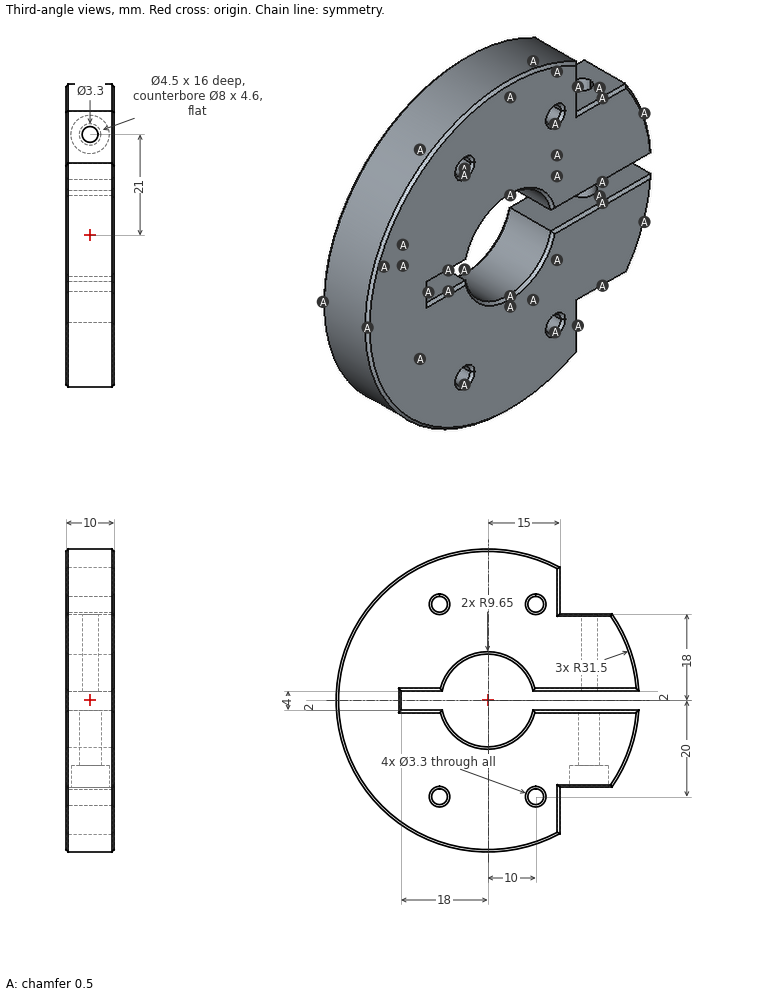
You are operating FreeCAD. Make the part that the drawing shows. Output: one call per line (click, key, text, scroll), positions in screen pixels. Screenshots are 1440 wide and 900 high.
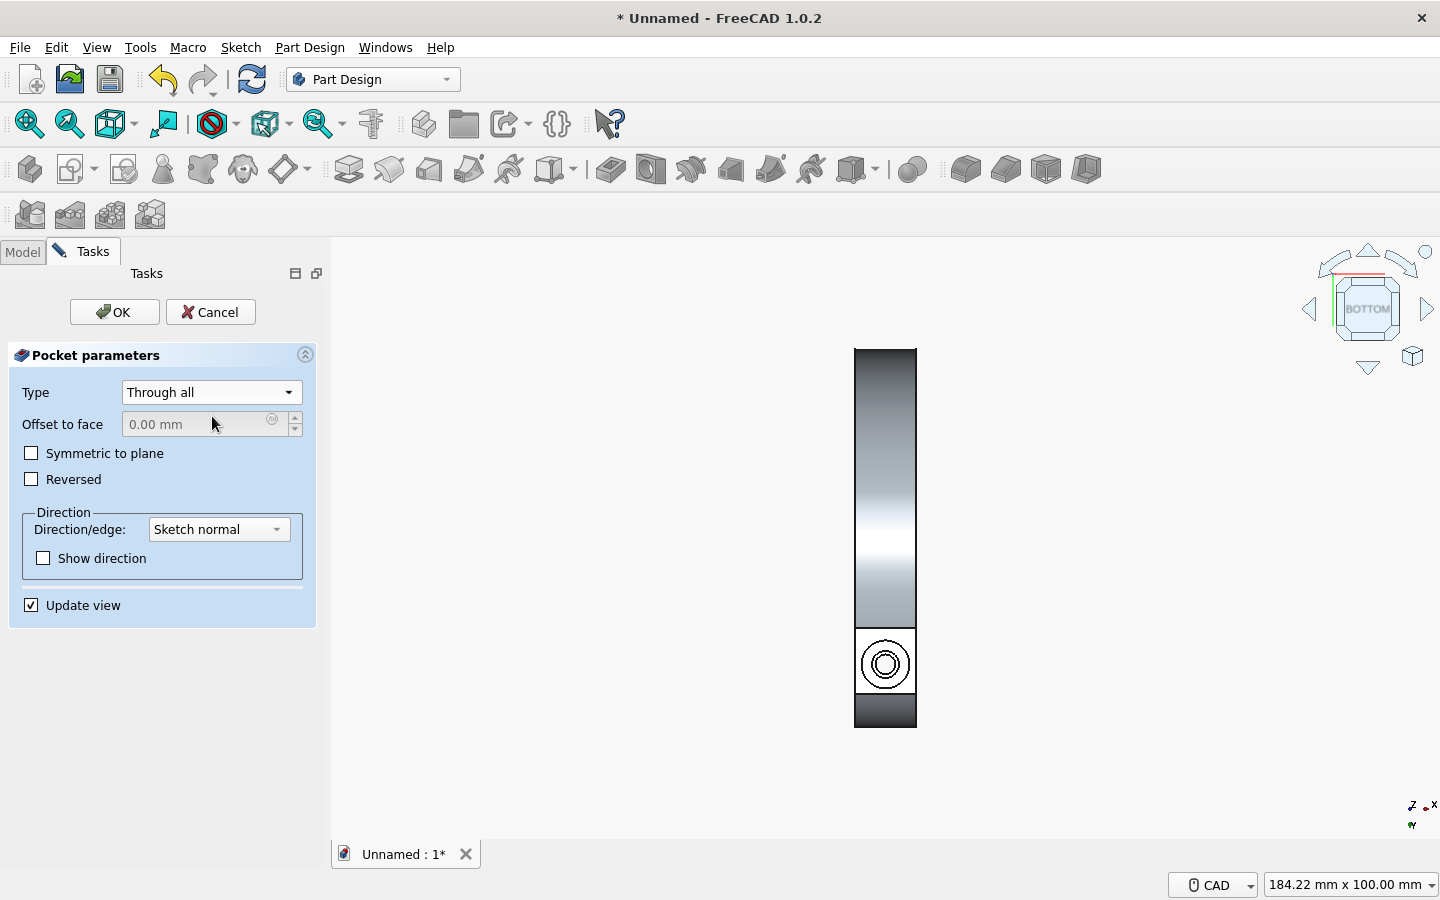
click(115, 312)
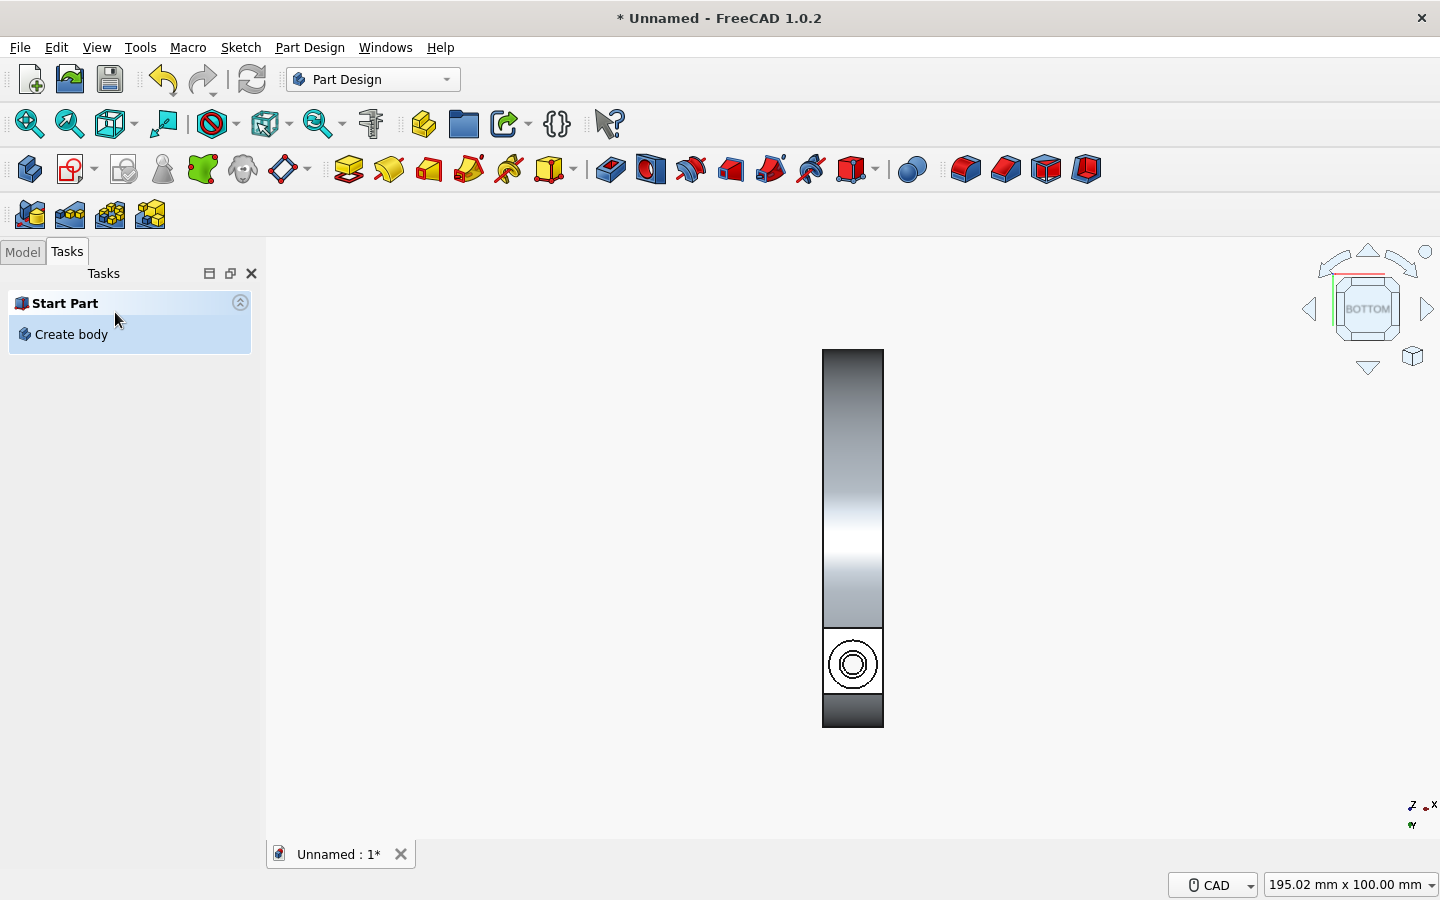
key(0)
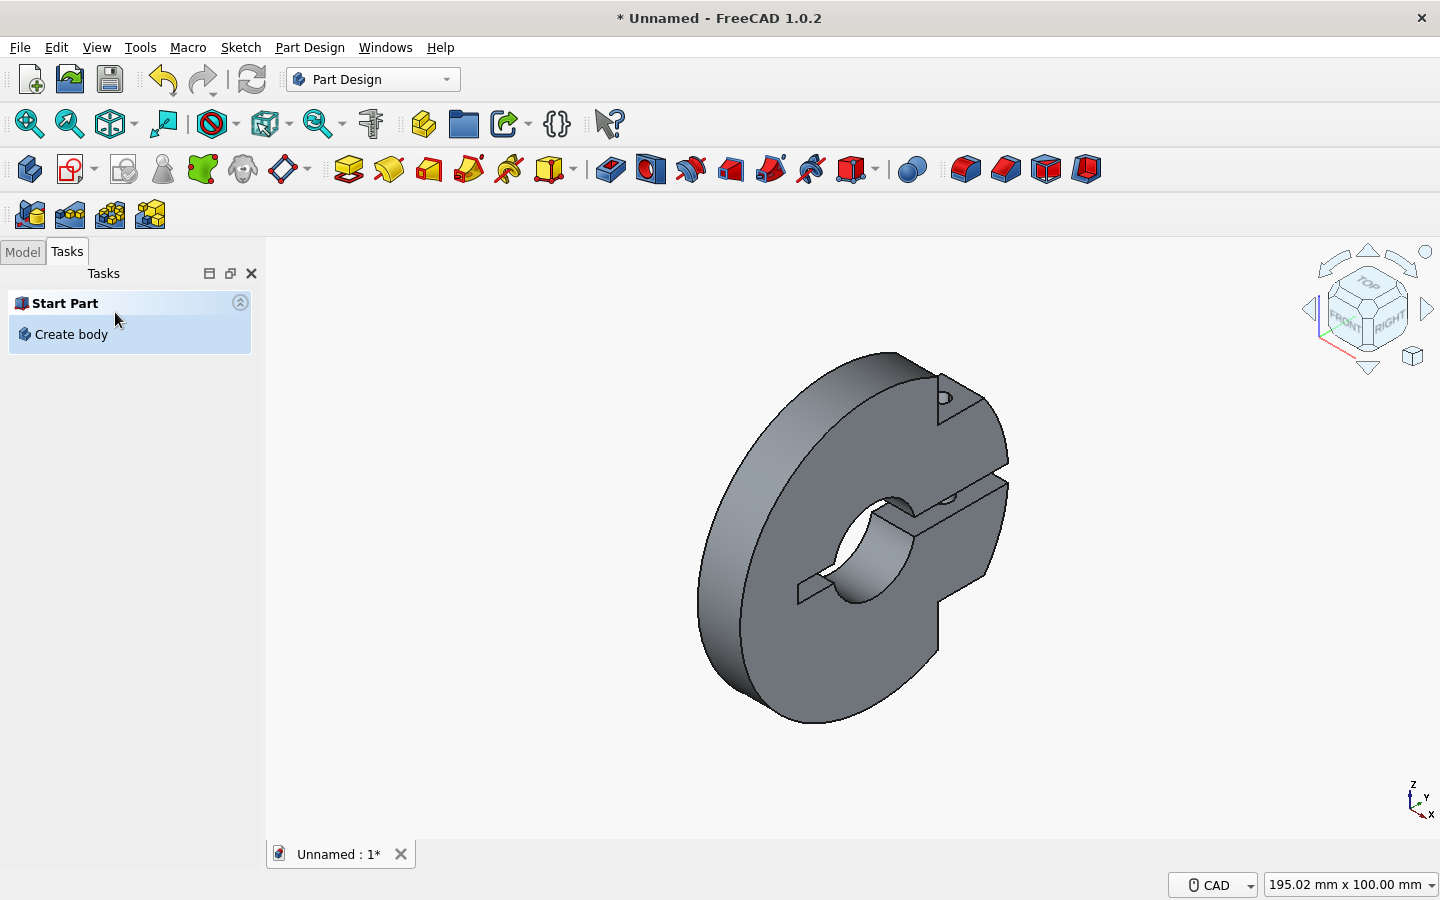
click(836, 483)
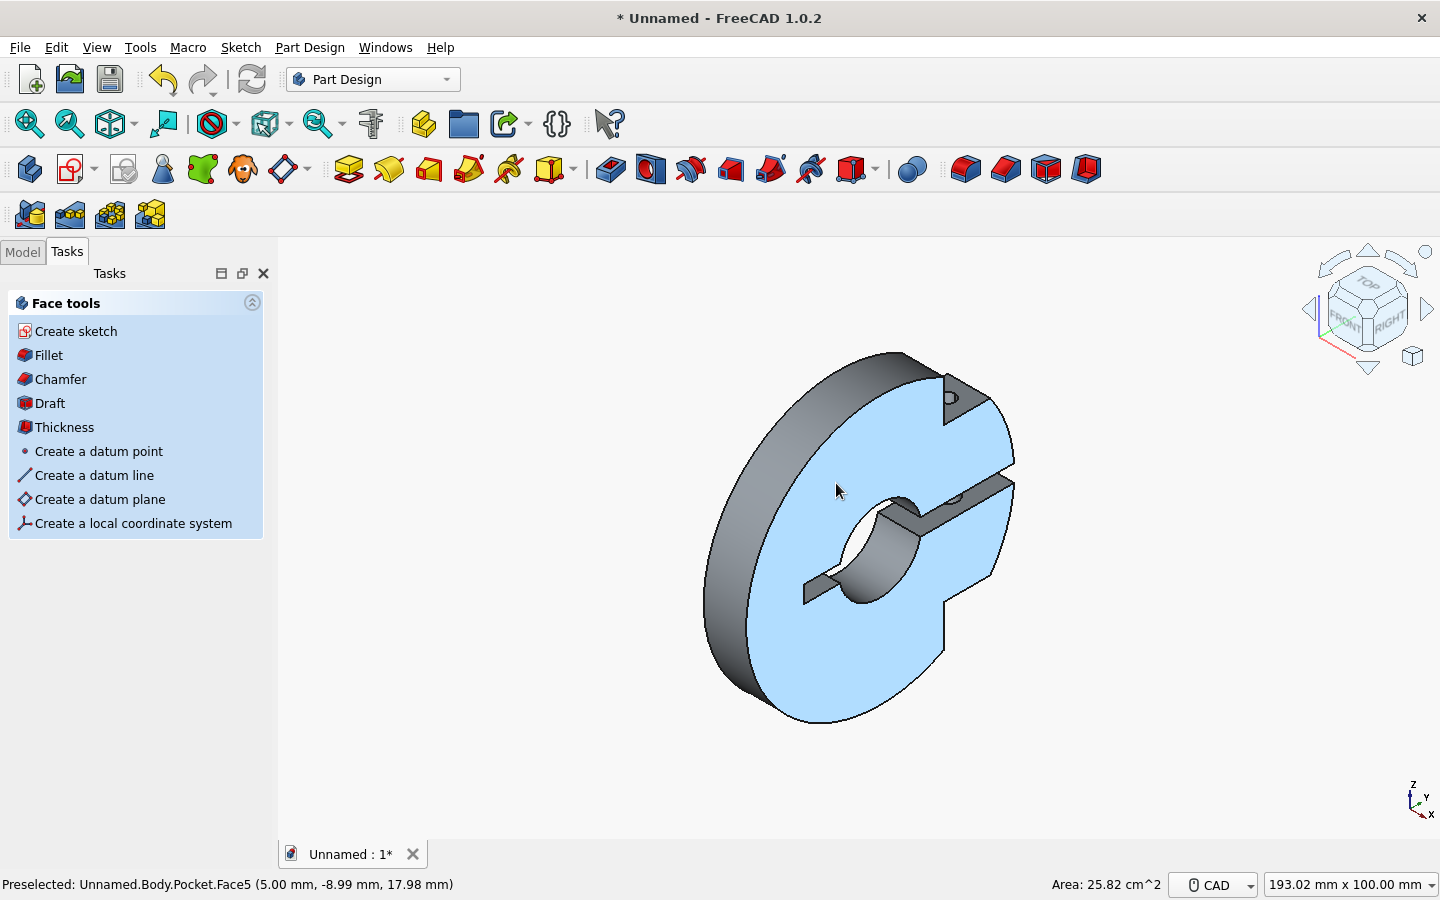
click(70, 170)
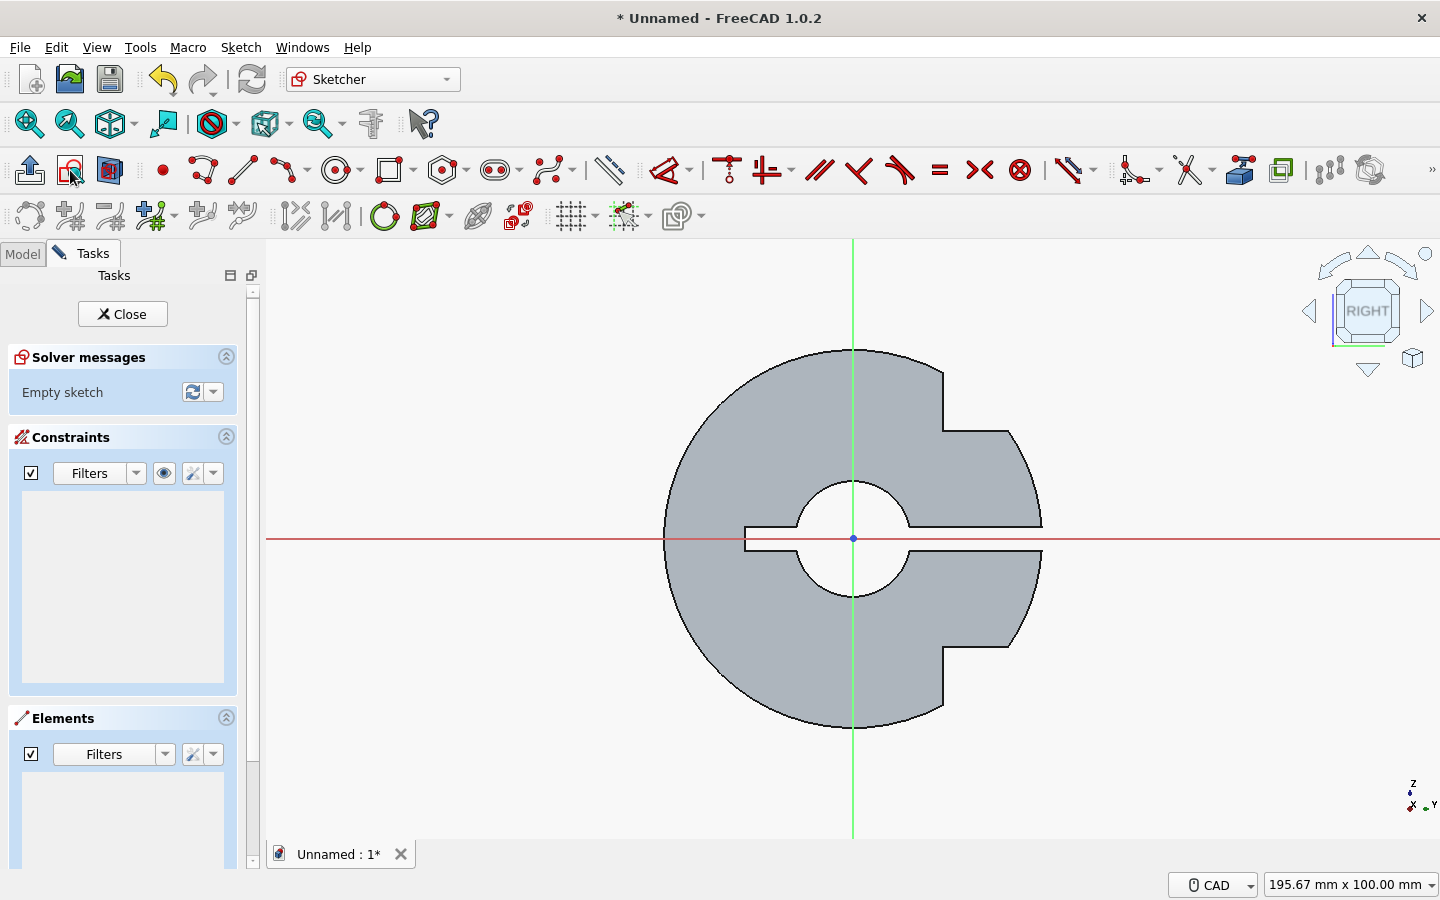
scroll(992, 539, up, 2)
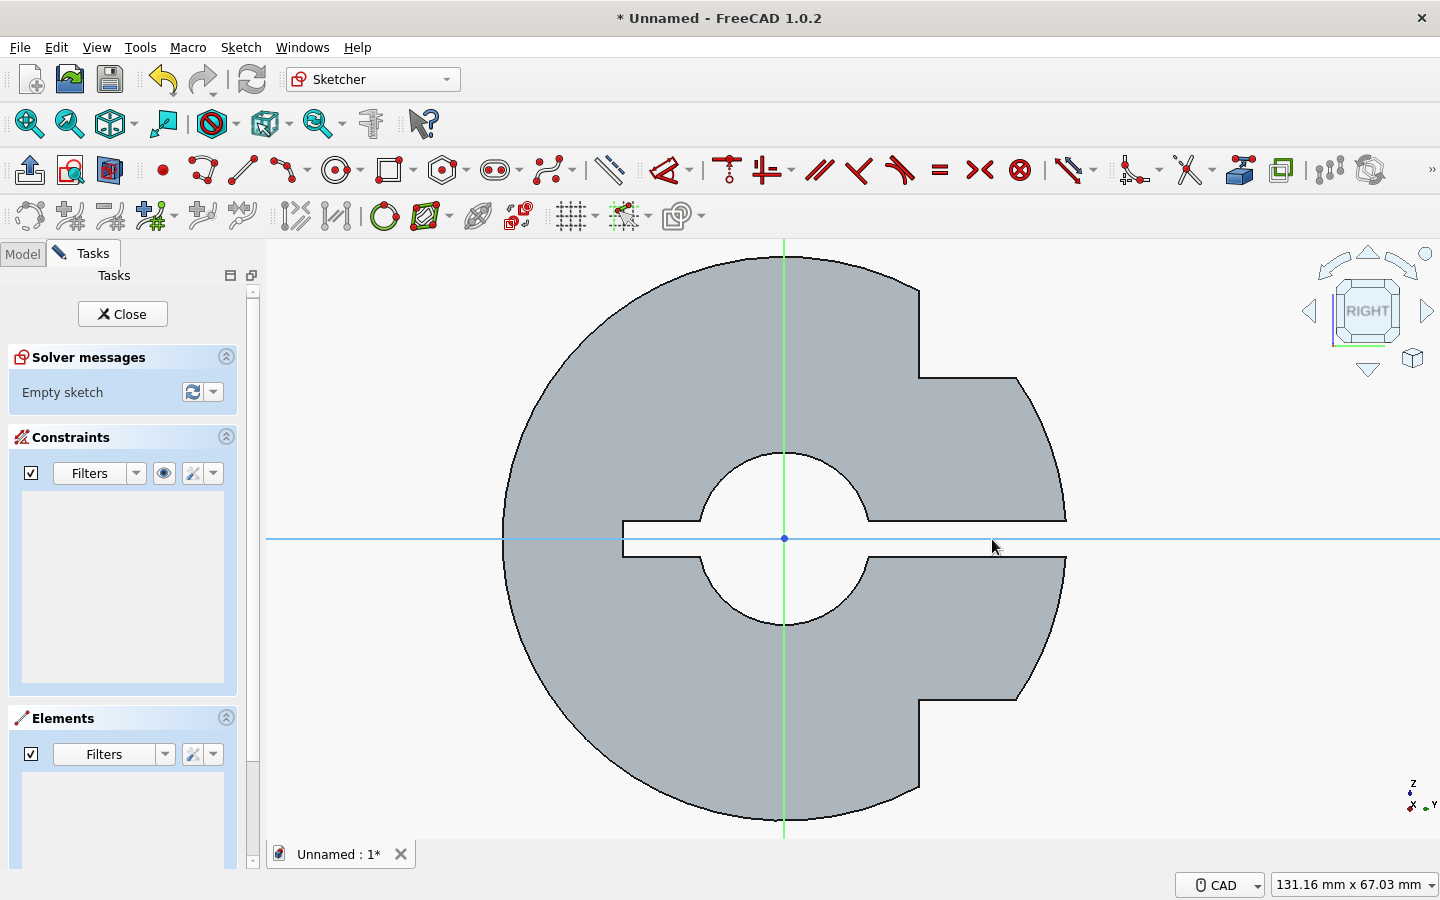
key(g)
key(c)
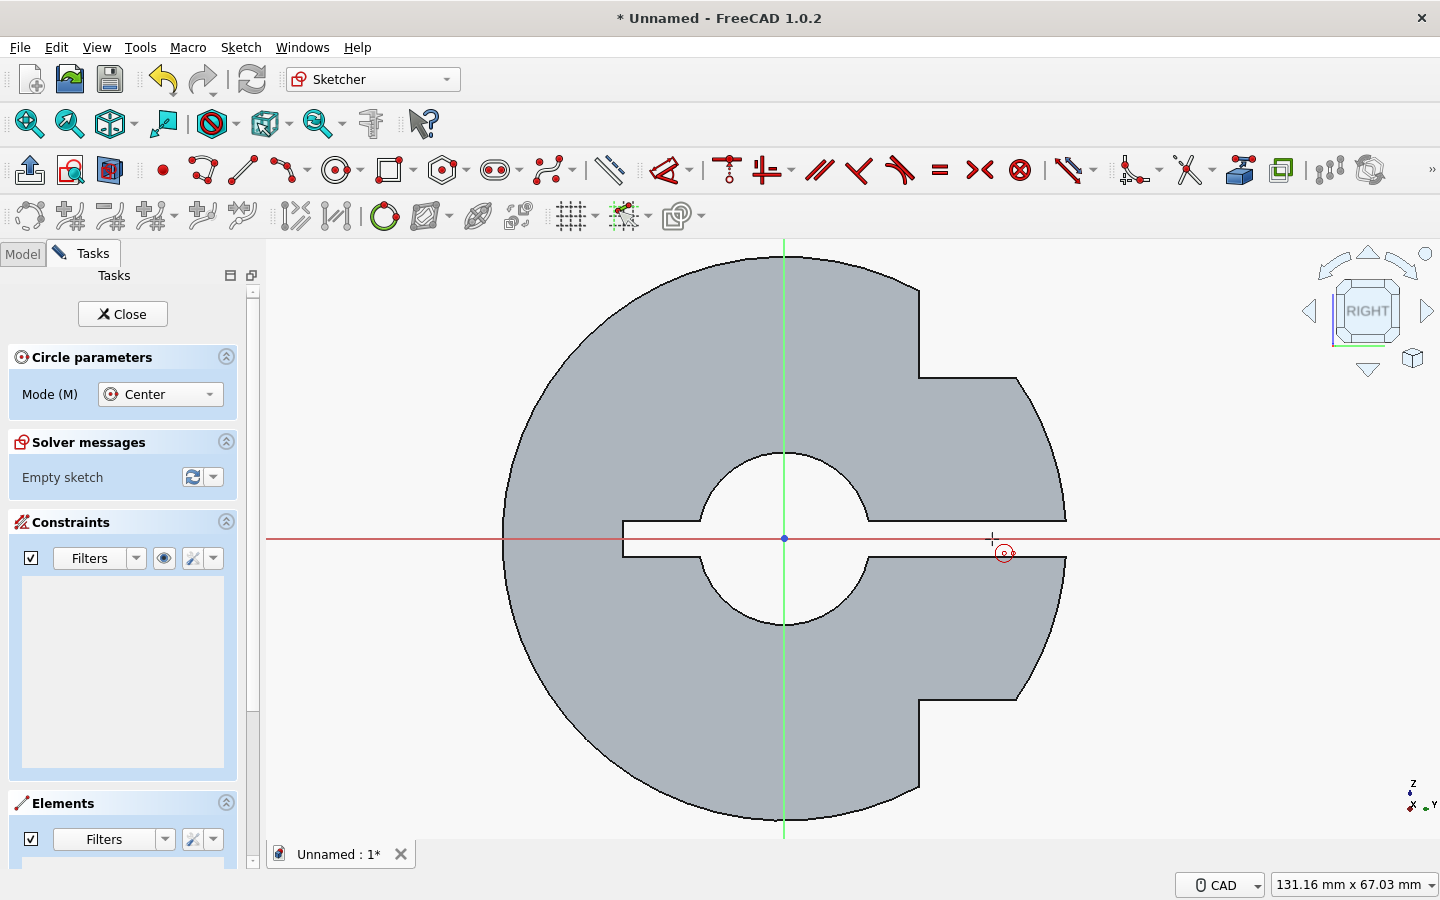
scroll(874, 718, up, 3)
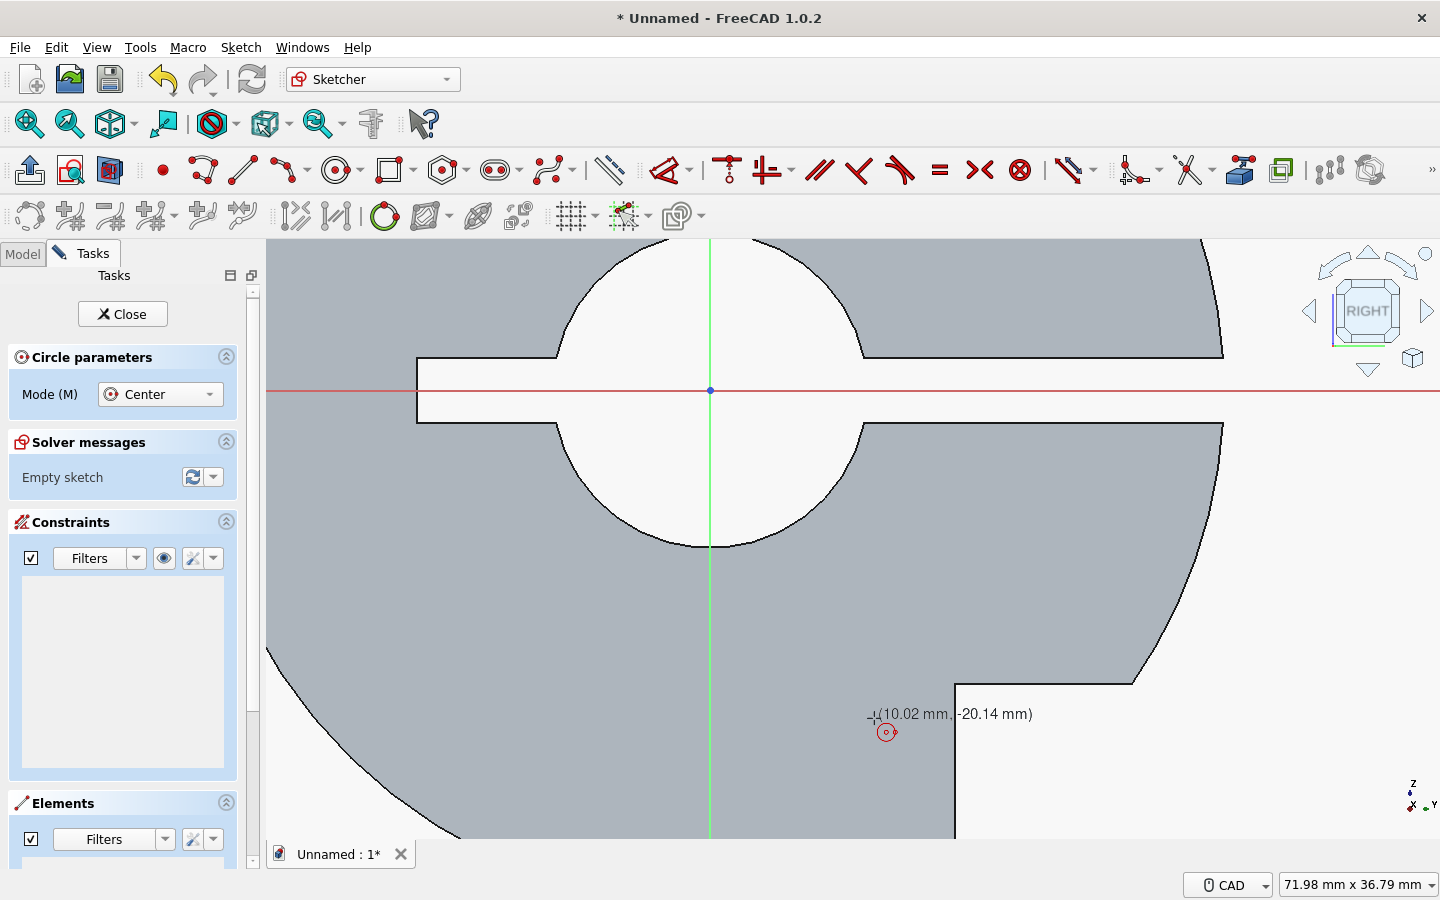
click(873, 717)
click(892, 698)